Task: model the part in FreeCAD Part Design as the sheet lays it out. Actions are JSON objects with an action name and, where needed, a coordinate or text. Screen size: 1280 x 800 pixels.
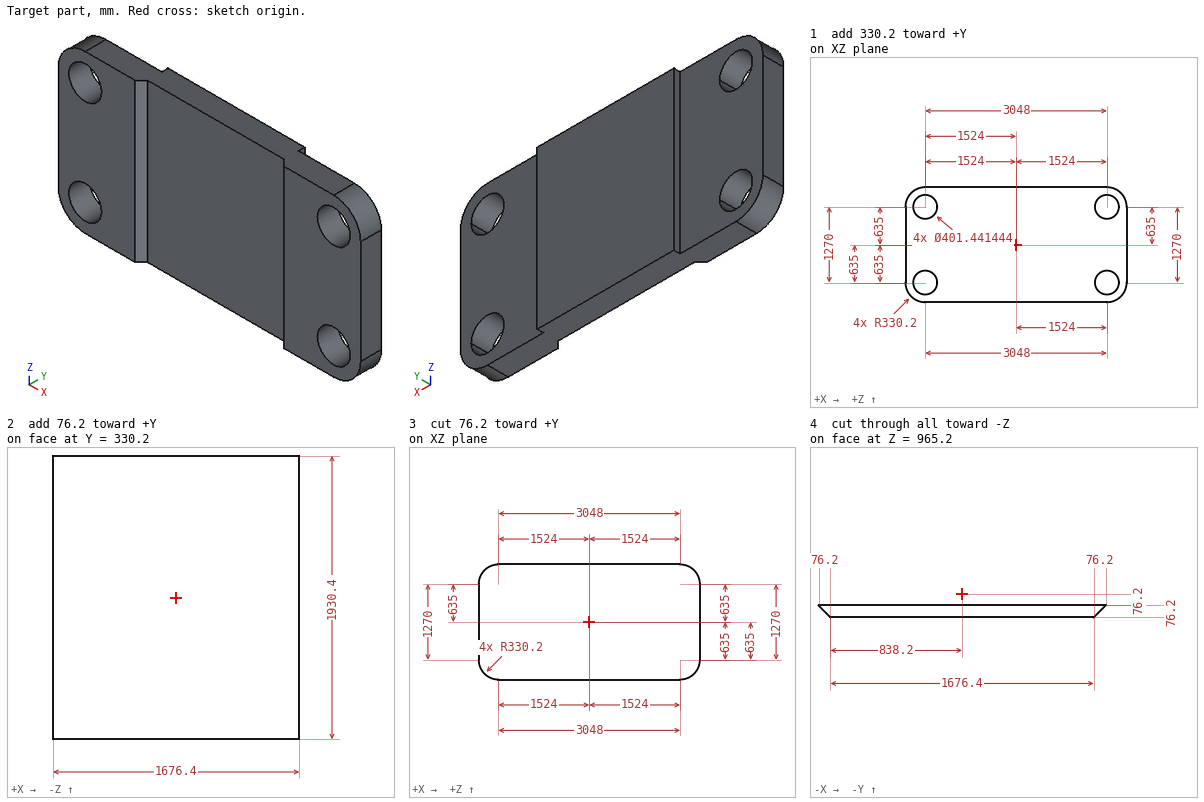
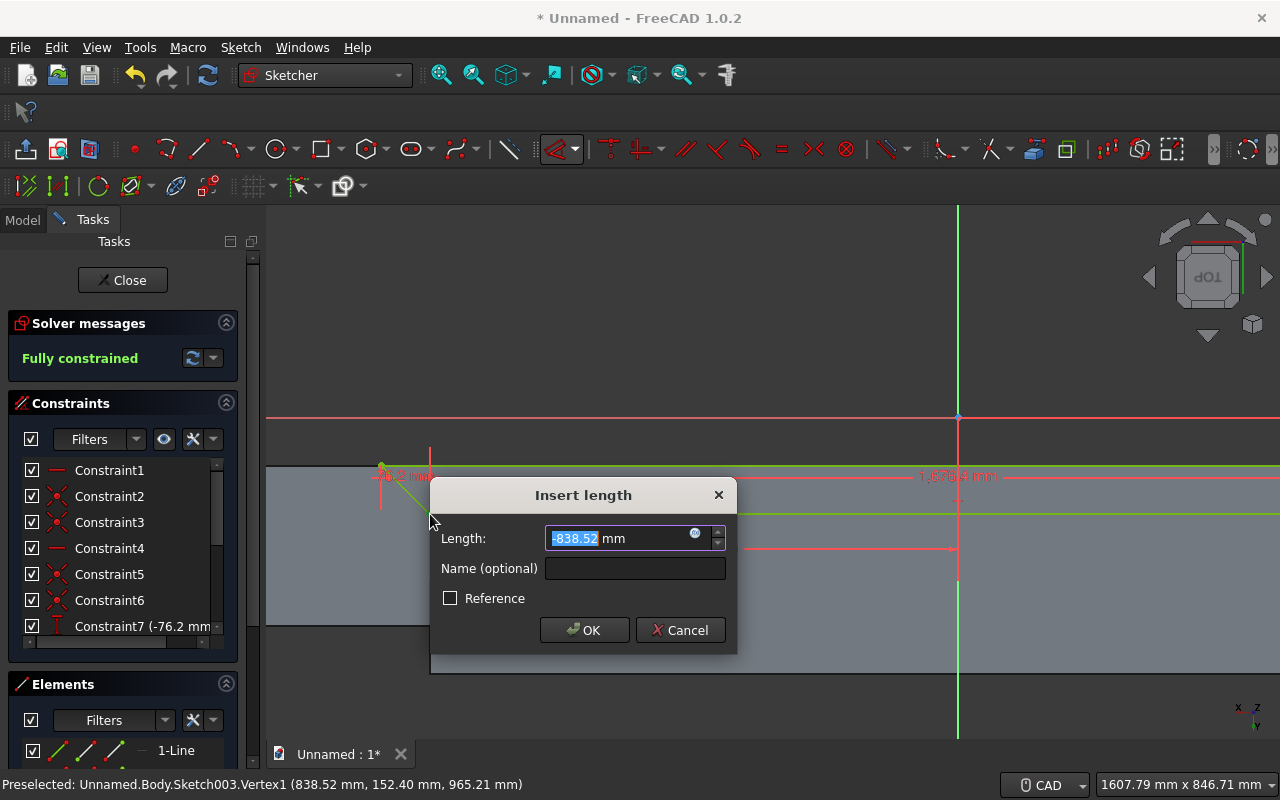
{"action": "type", "text": "-838.2"}
{"action": "key", "text": "Return"}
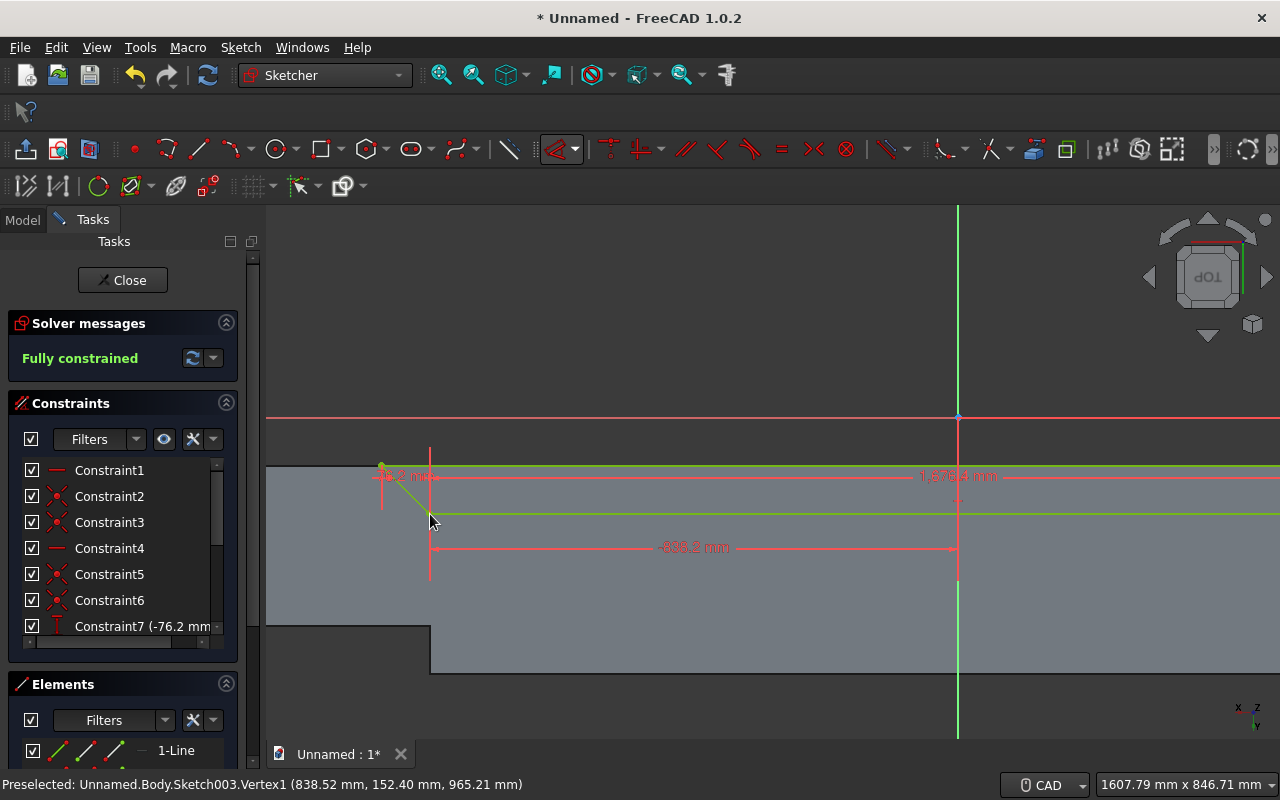
{"action": "left_click", "coordinate": [123, 280]}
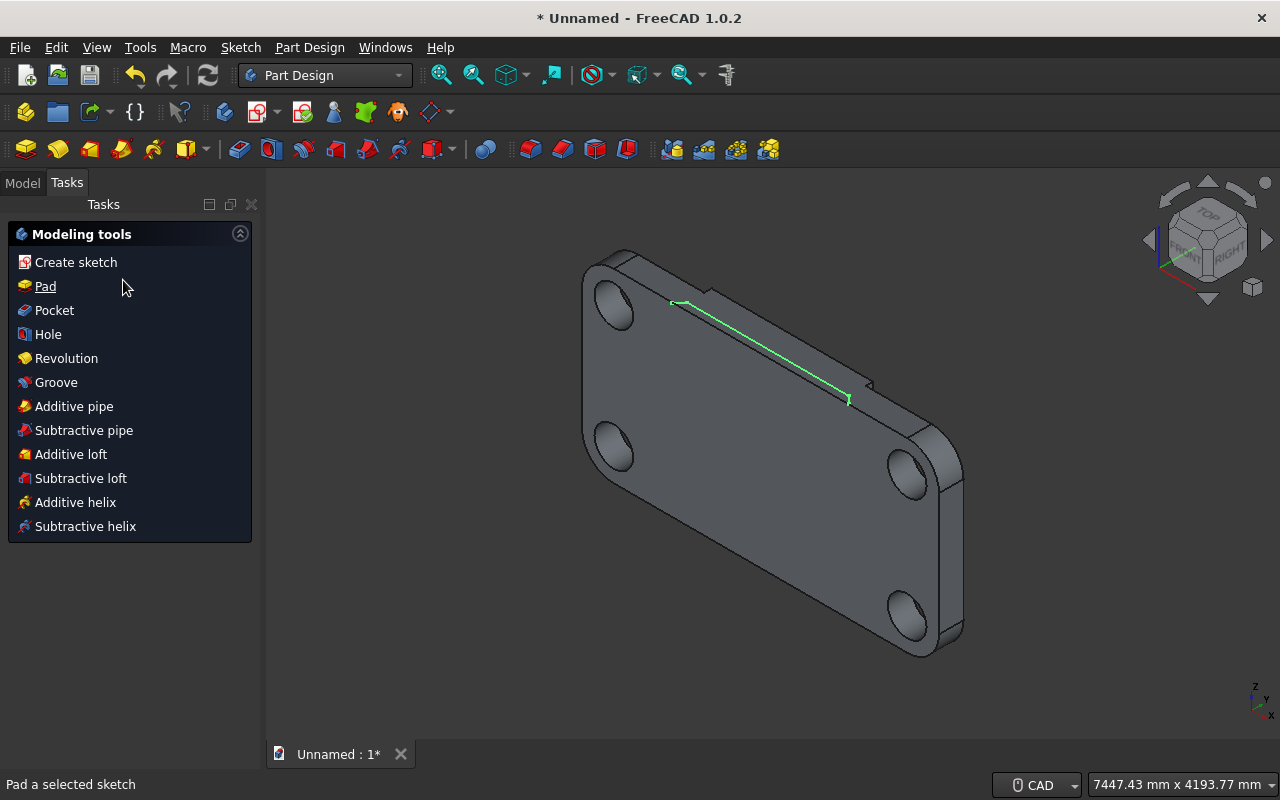
{"action": "left_click", "coordinate": [240, 150]}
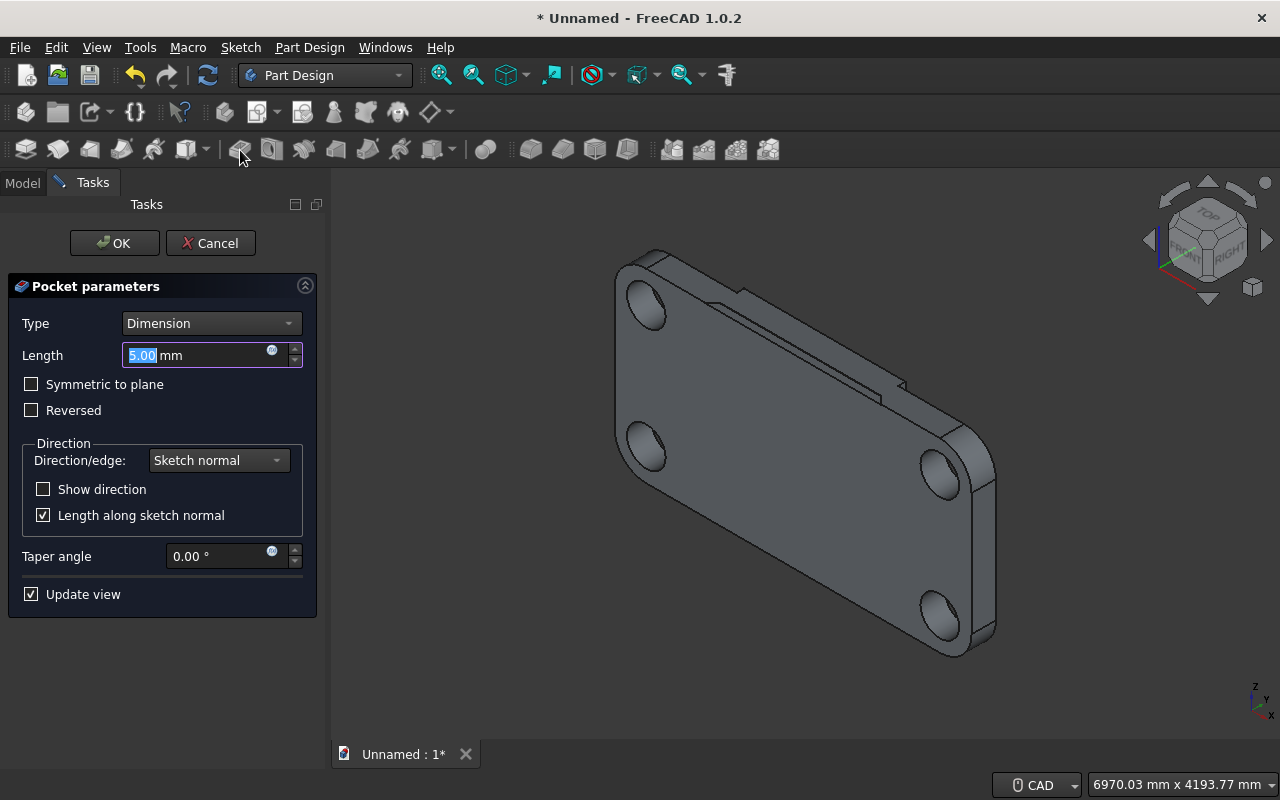
{"action": "left_click", "coordinate": [212, 324]}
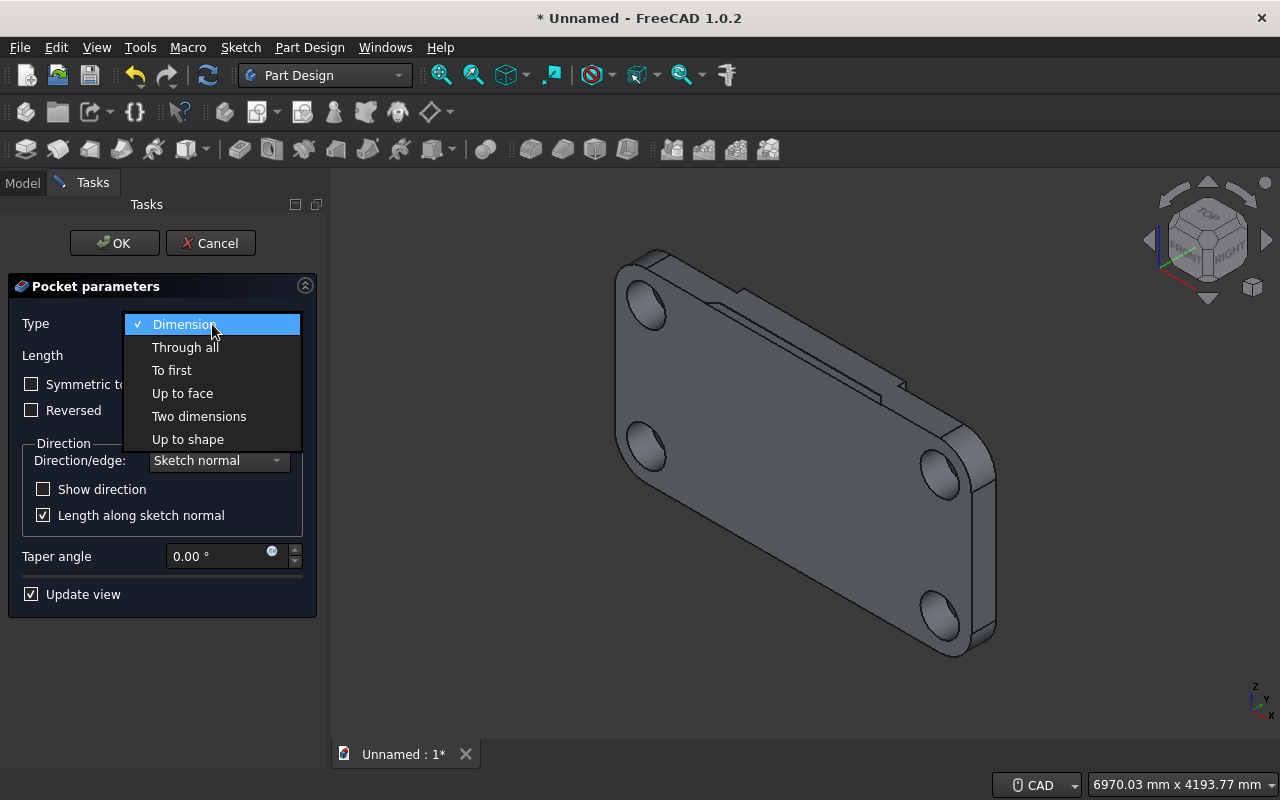
{"action": "left_click", "coordinate": [212, 348]}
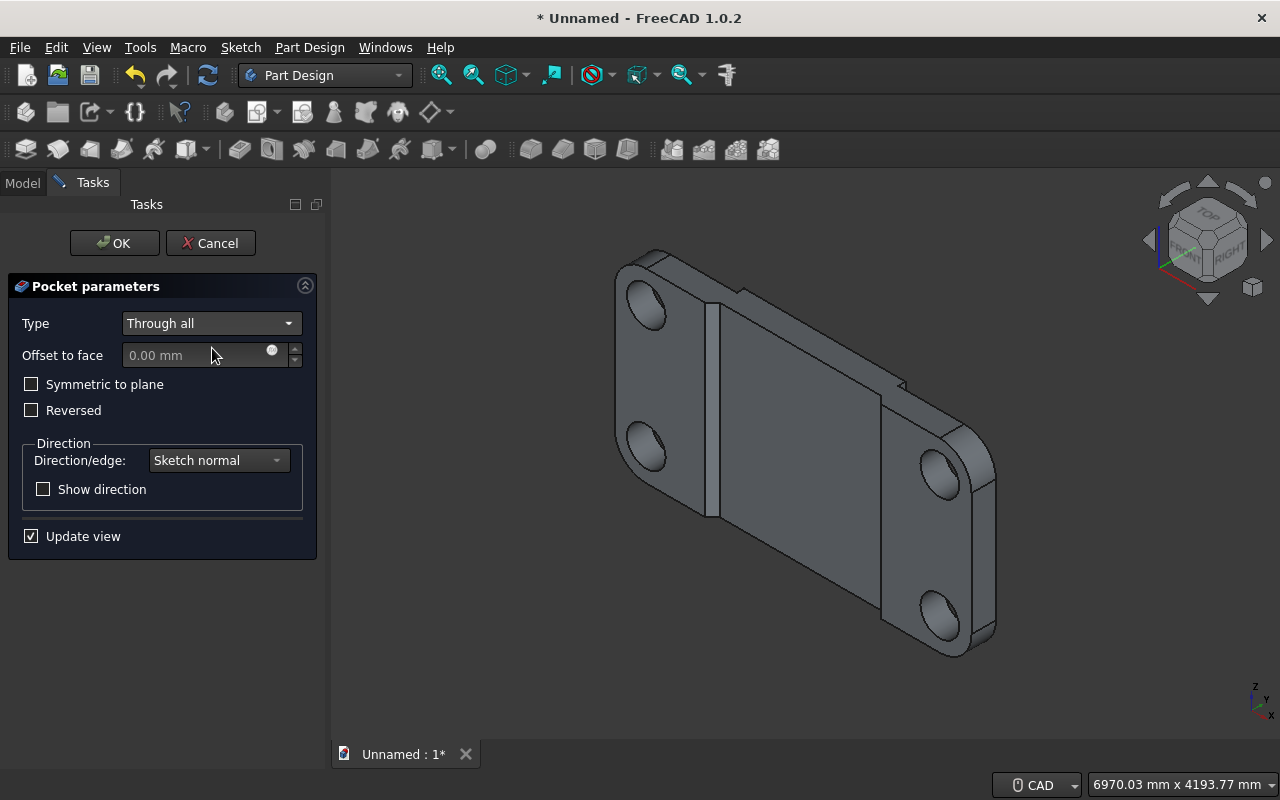
{"action": "left_click", "coordinate": [115, 243]}